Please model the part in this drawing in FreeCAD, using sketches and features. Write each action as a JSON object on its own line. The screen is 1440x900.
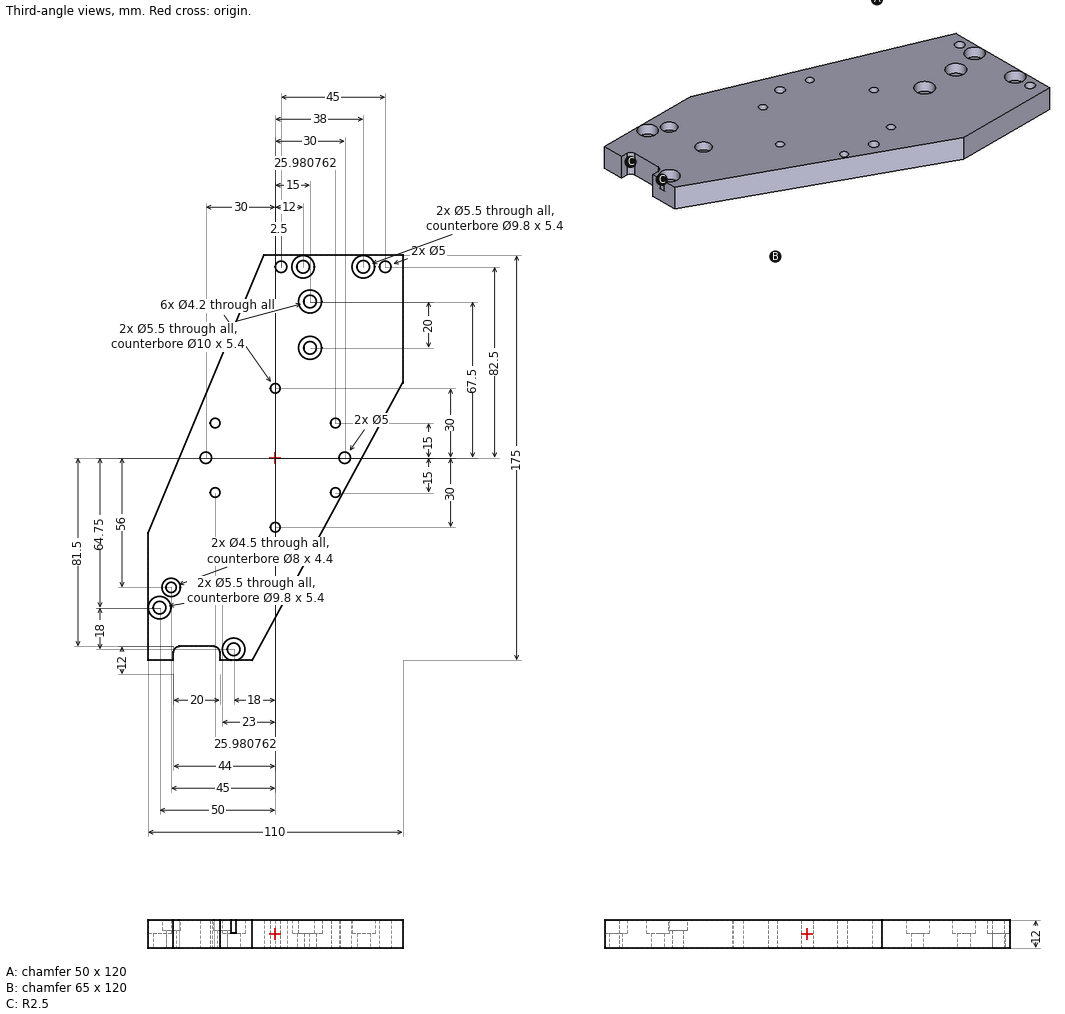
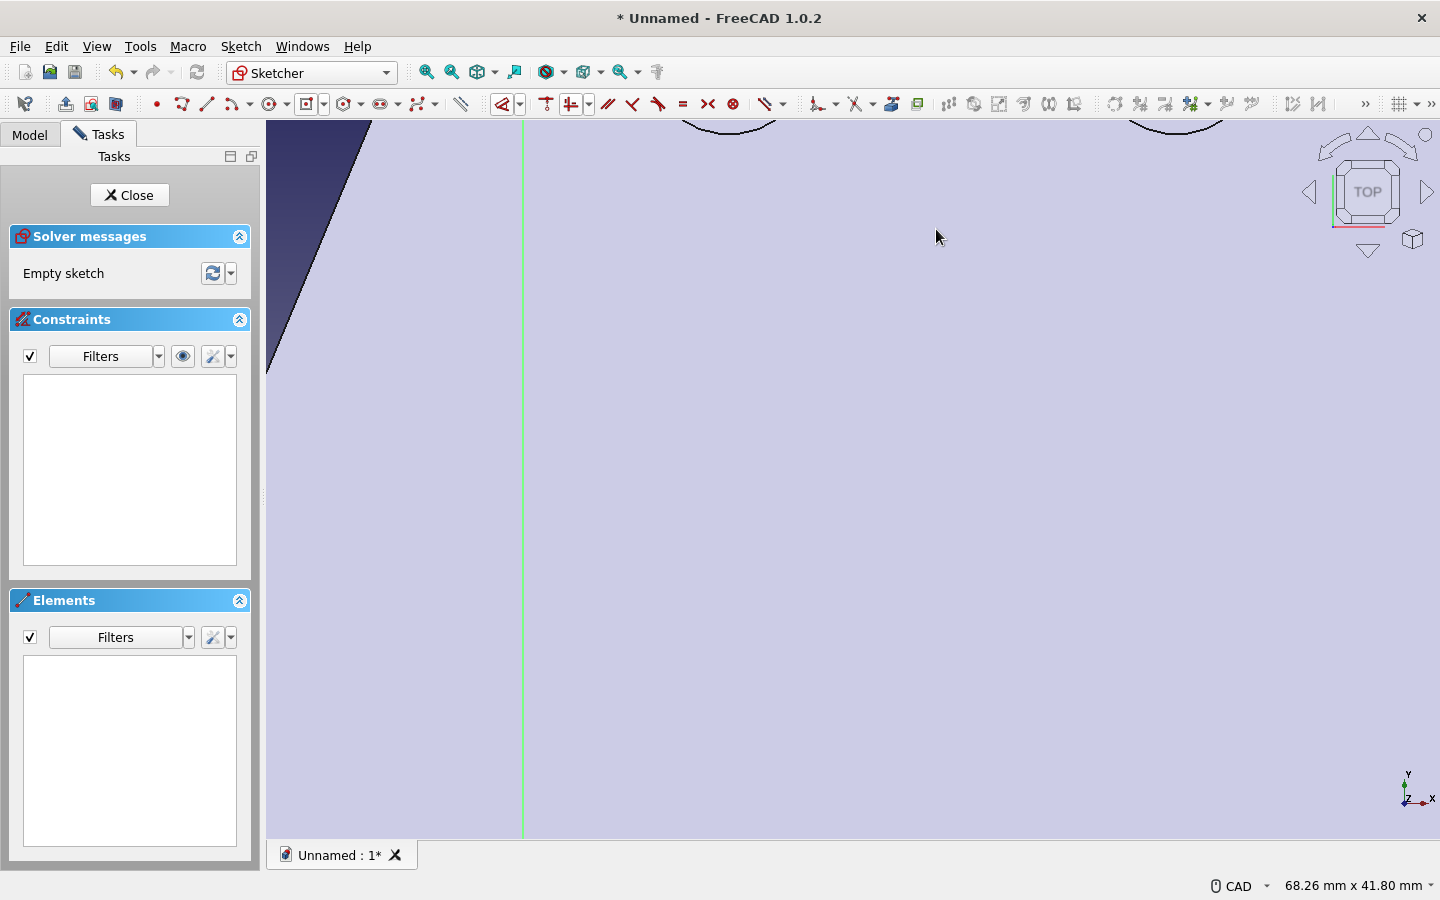
{"action": "left_click", "coordinate": [268, 104]}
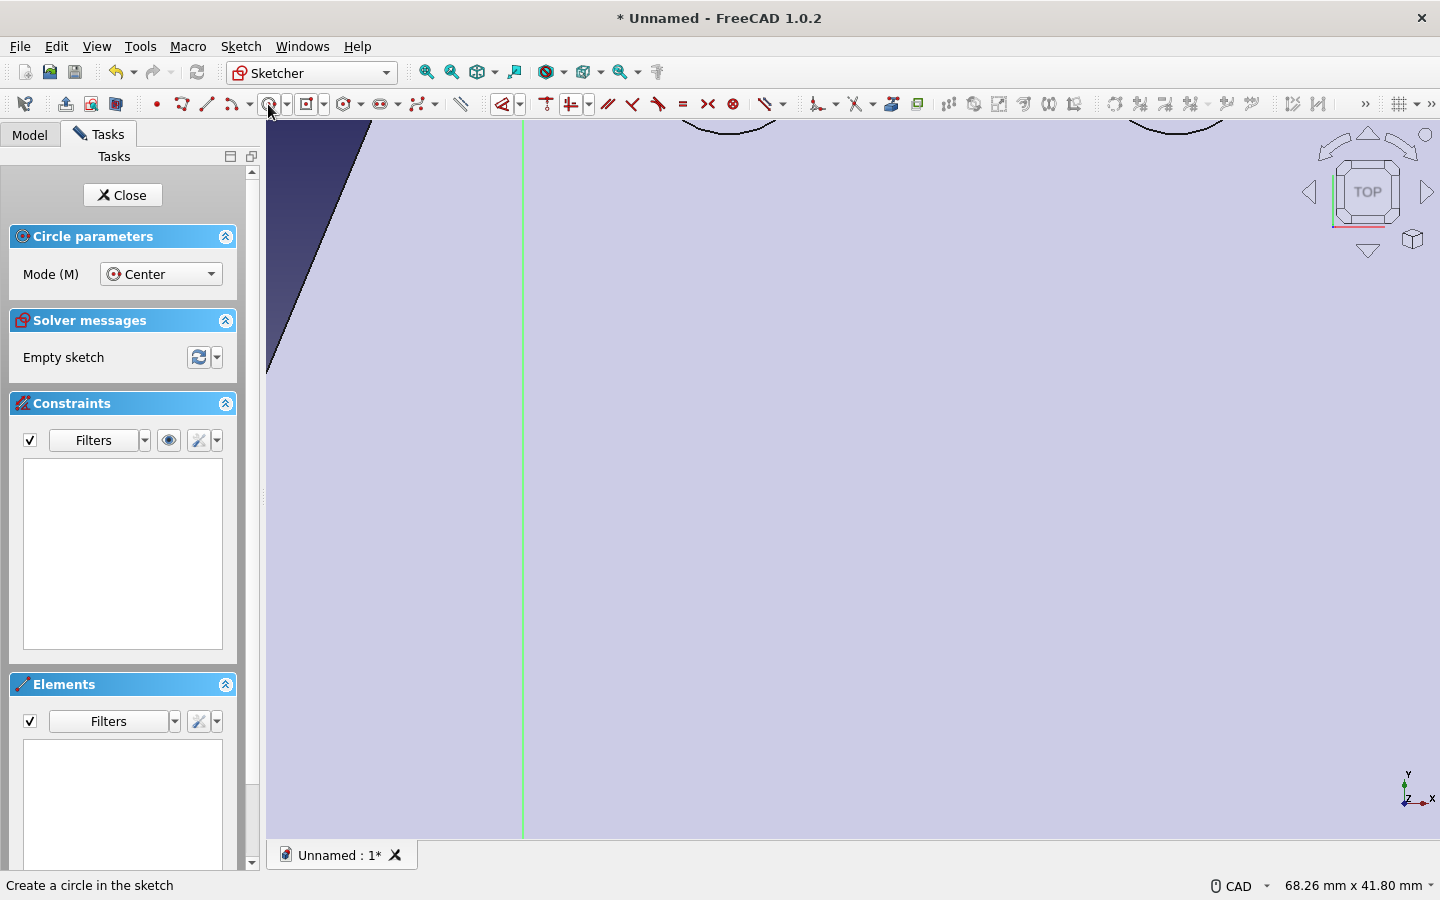
{"action": "left_click", "coordinate": [781, 308]}
{"action": "left_click", "coordinate": [814, 275]}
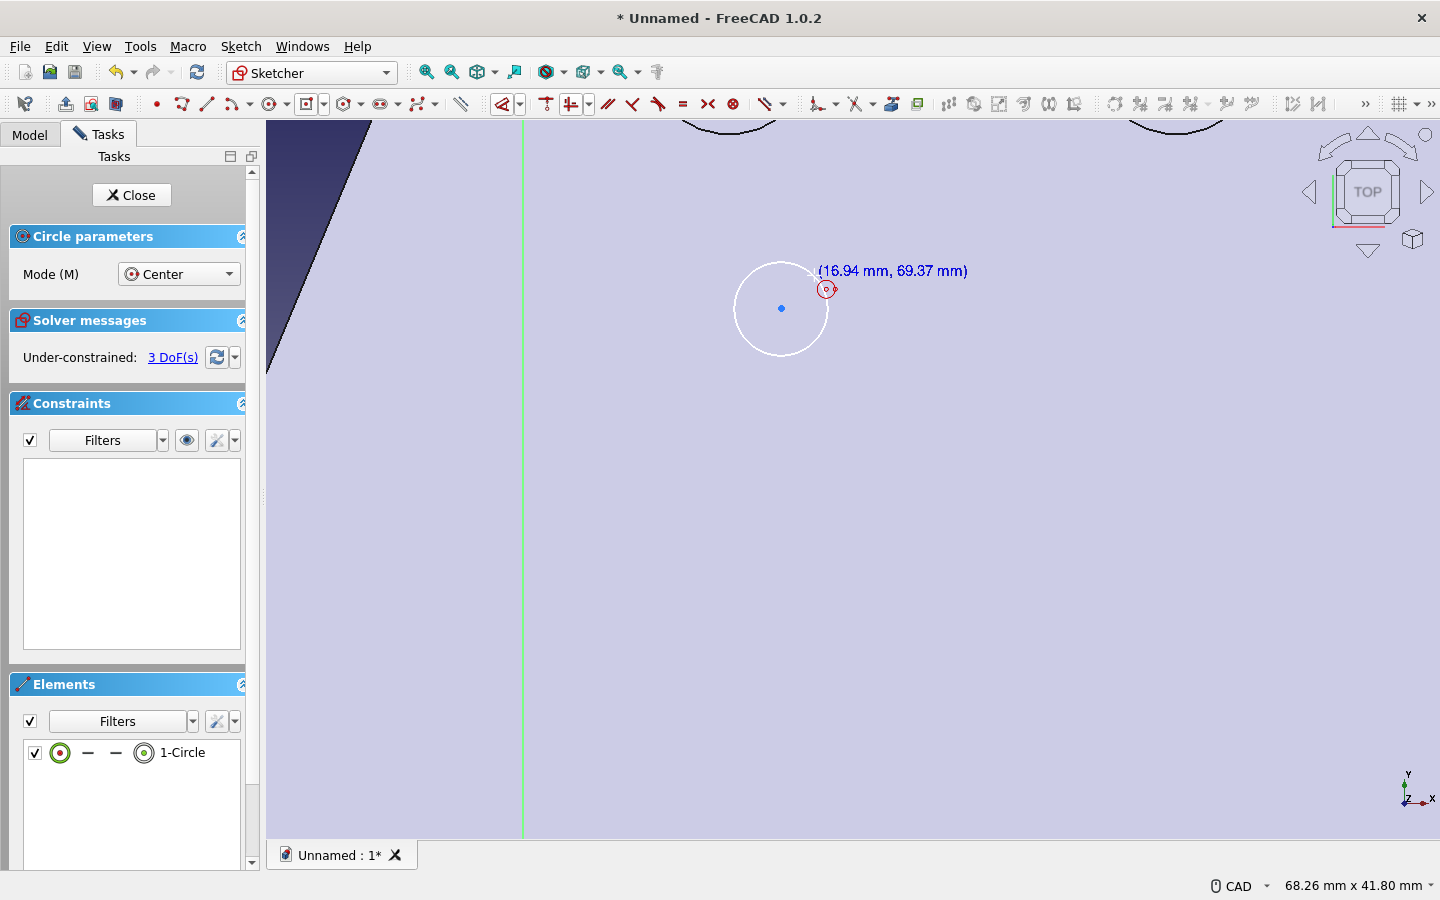
{"action": "left_click", "coordinate": [781, 652]}
{"action": "left_click", "coordinate": [814, 619]}
{"action": "key", "text": "Escape"}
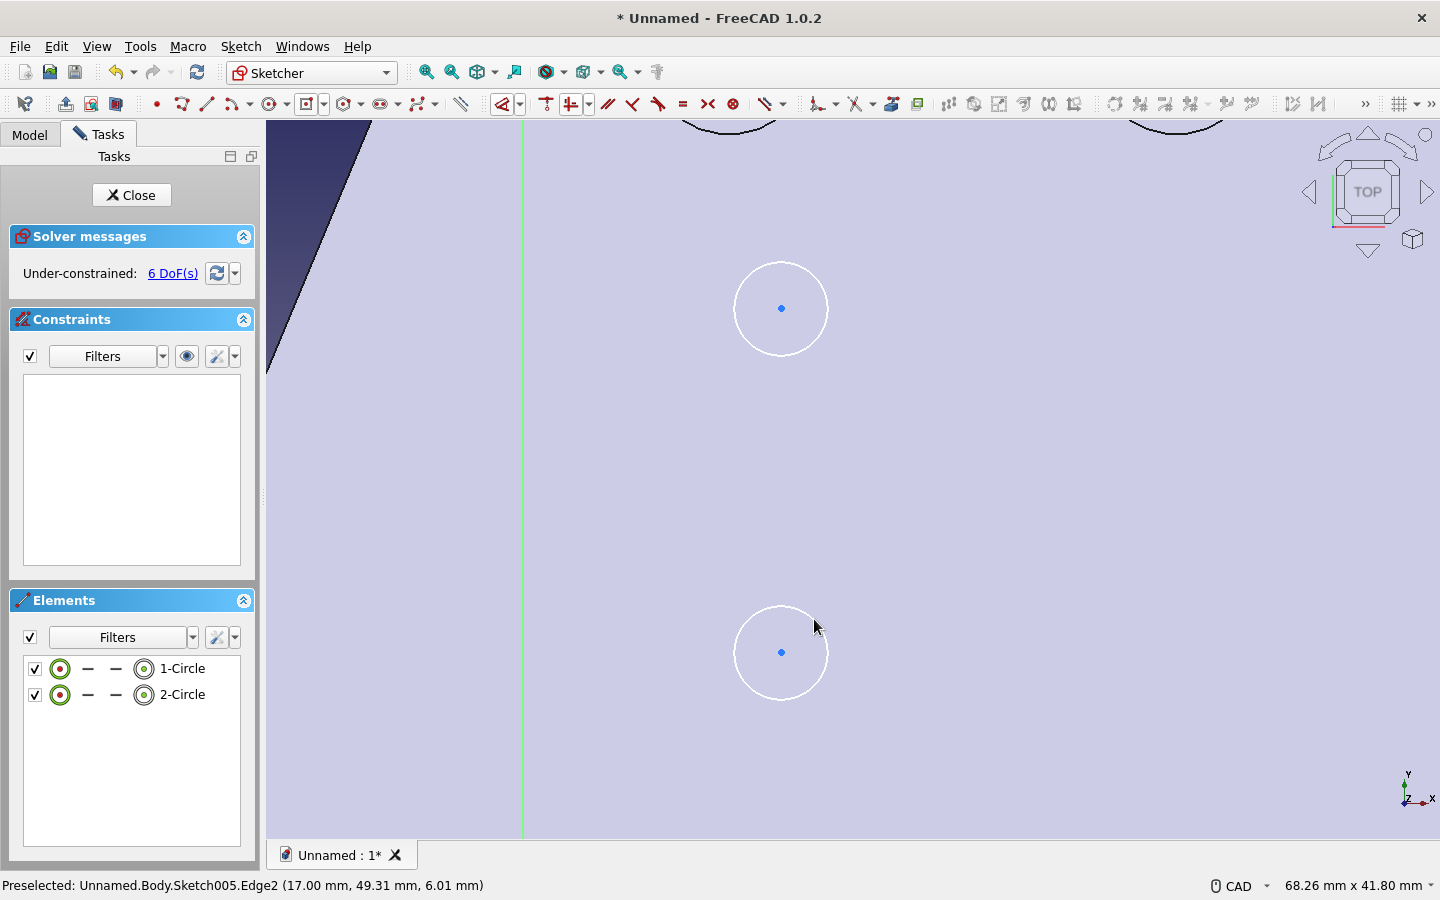
{"action": "left_click", "coordinate": [814, 276]}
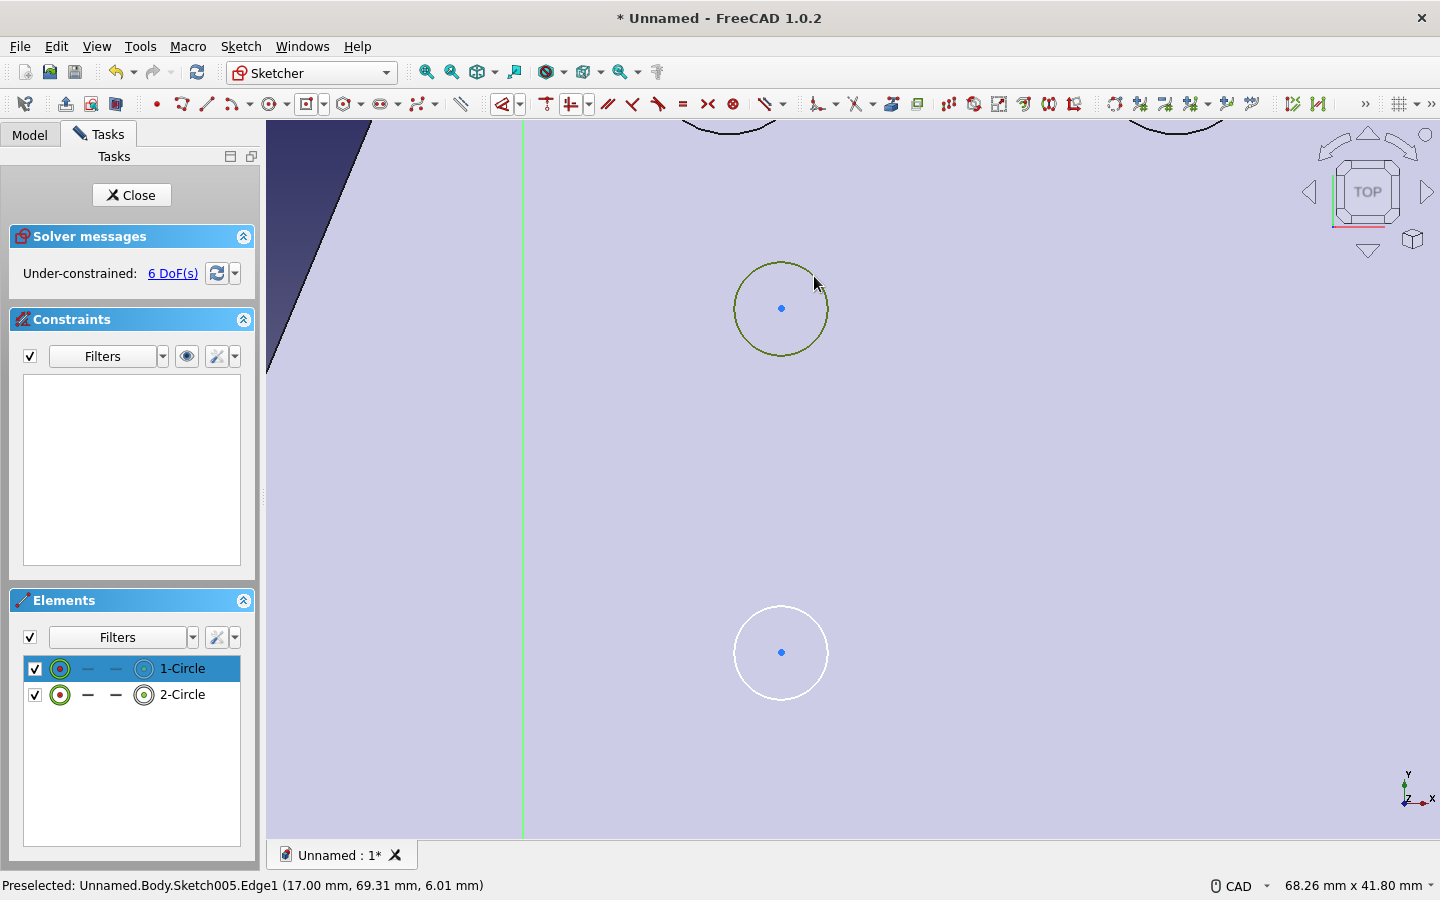
{"action": "left_click", "coordinate": [814, 620]}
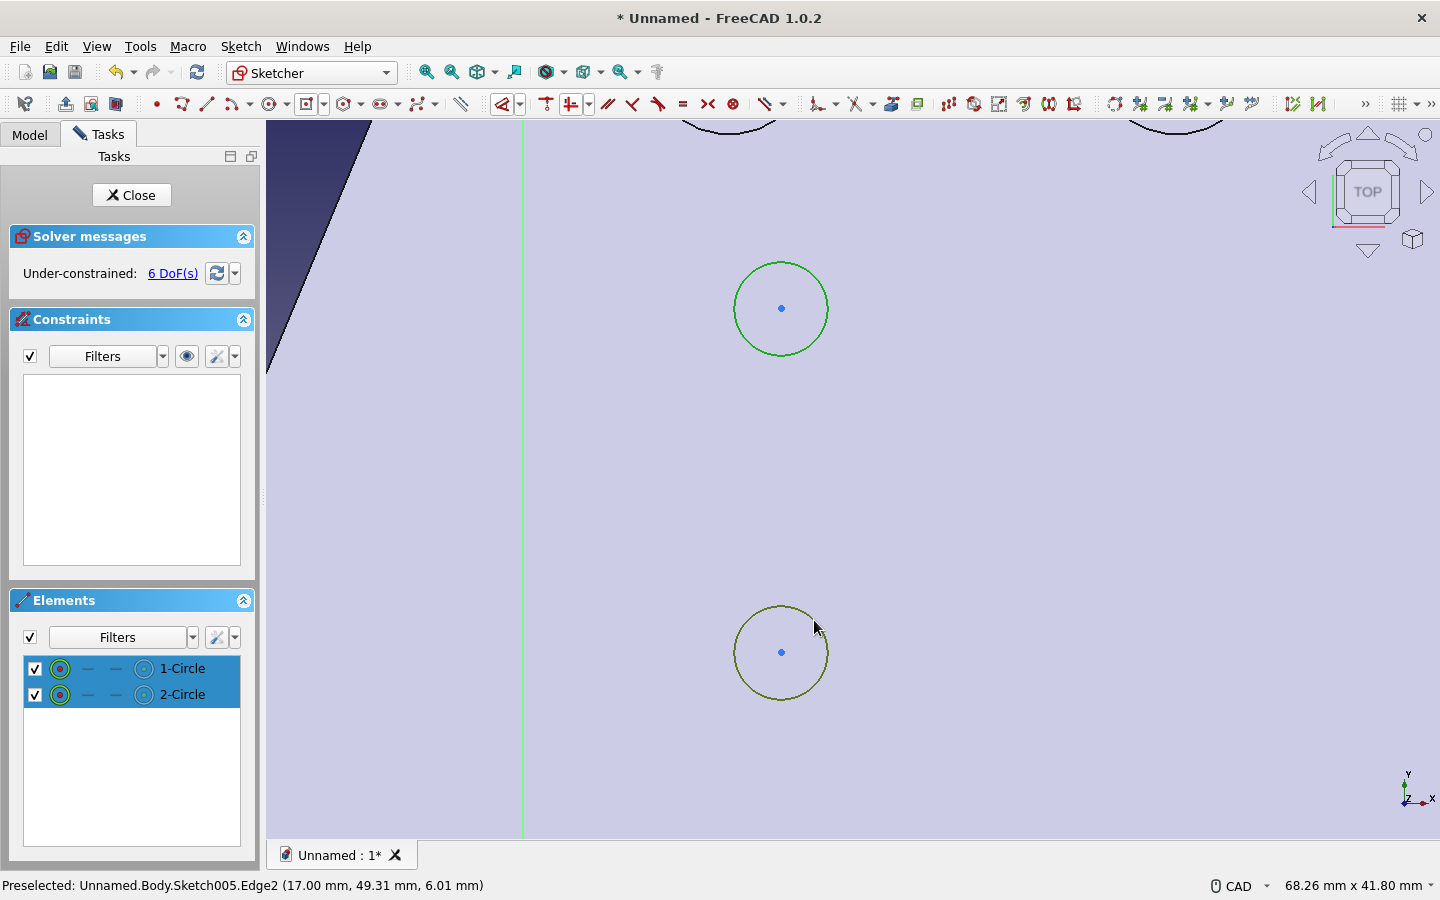
{"action": "left_click", "coordinate": [683, 104]}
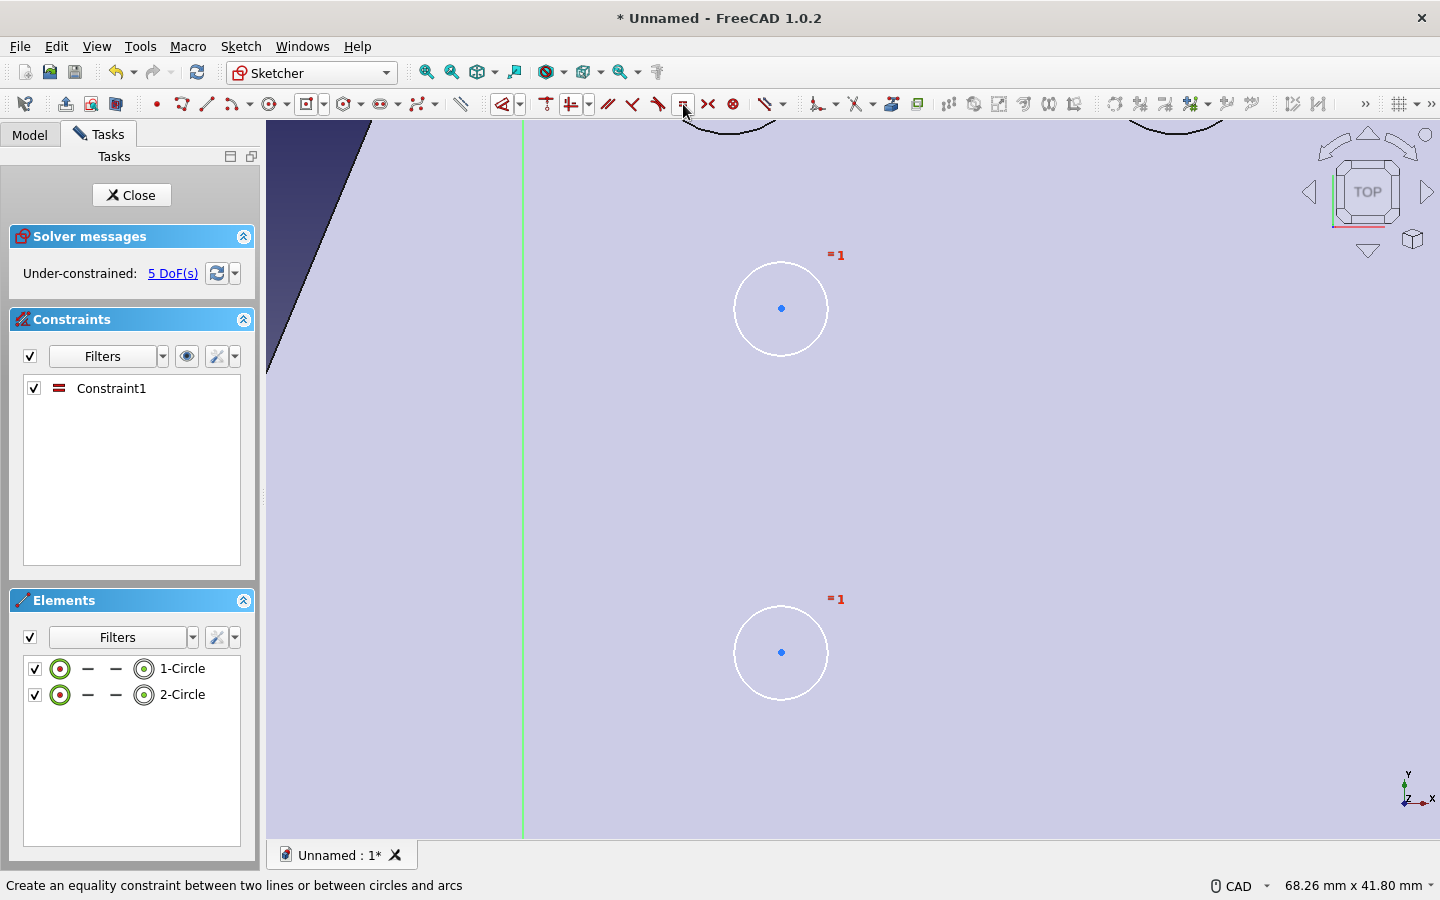
{"action": "left_click", "coordinate": [781, 309]}